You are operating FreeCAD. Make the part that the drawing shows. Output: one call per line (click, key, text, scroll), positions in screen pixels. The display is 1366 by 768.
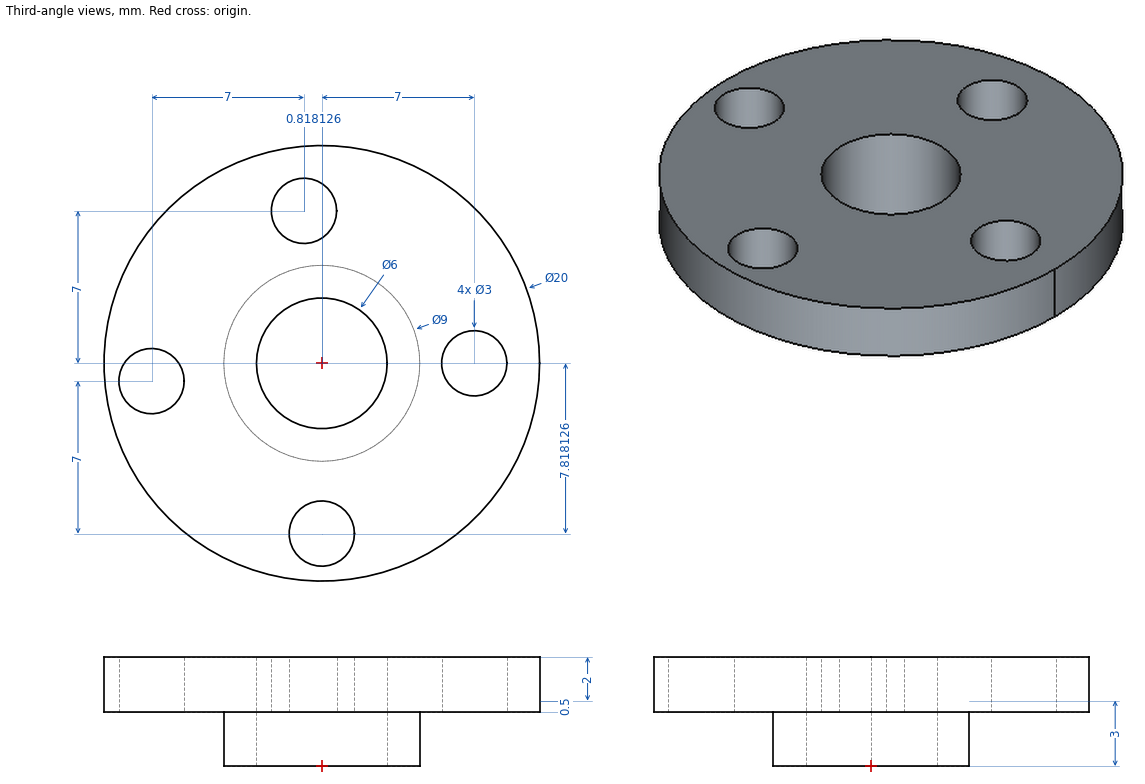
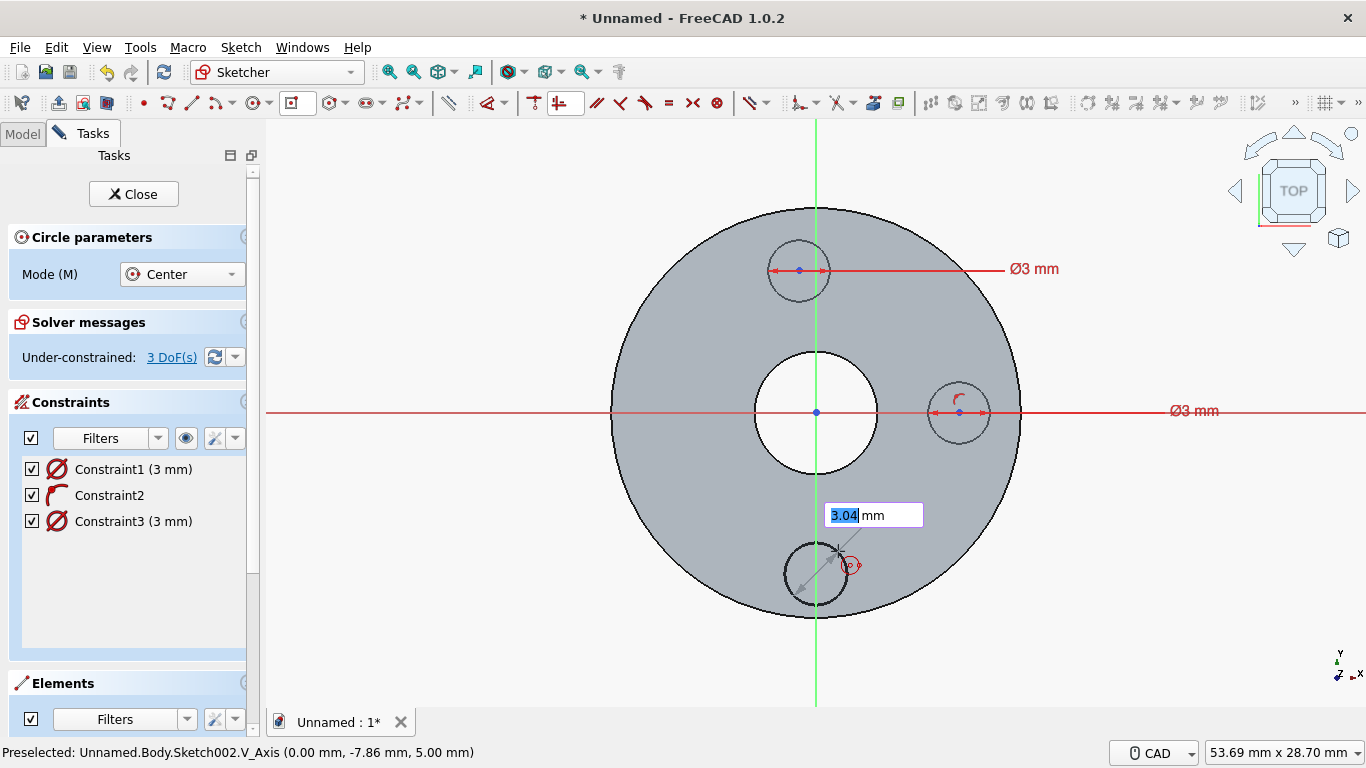
text(3)
key(Return)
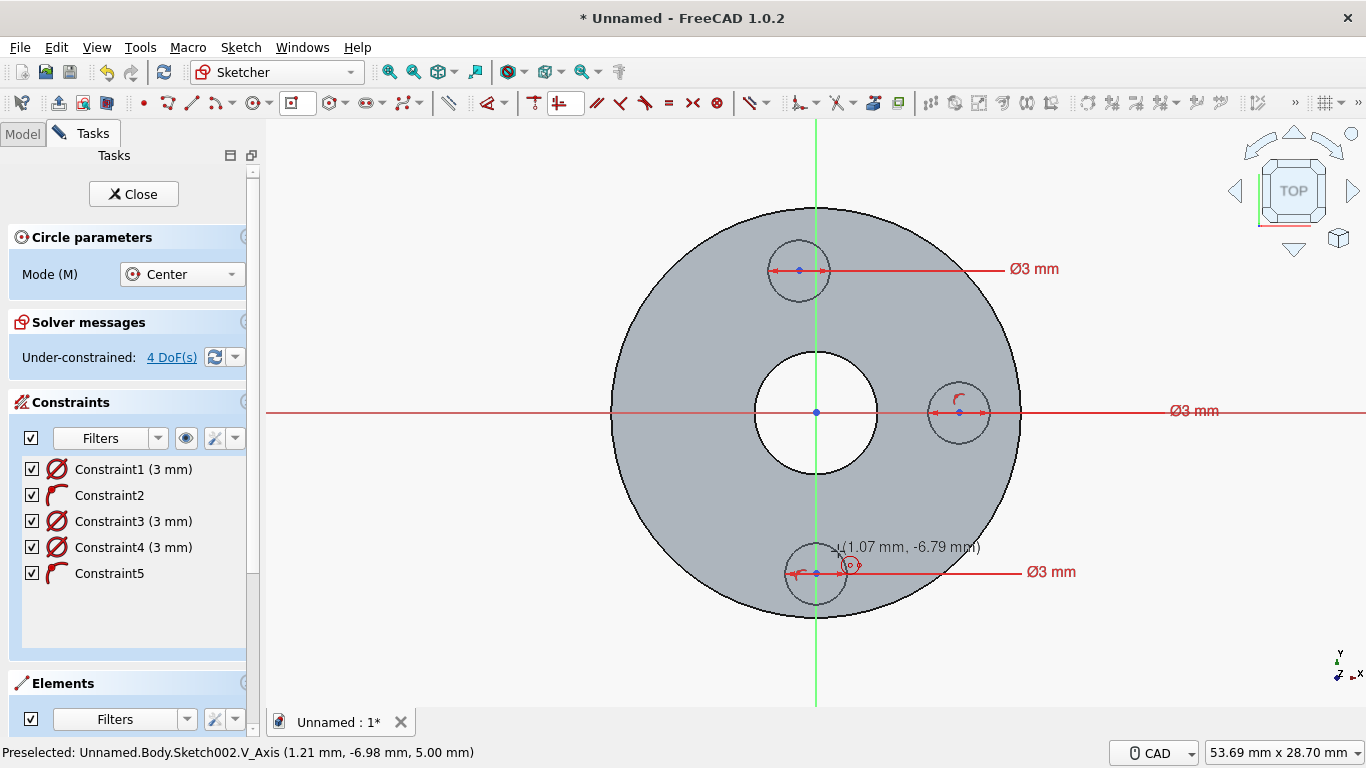
click(656, 430)
move(678, 451)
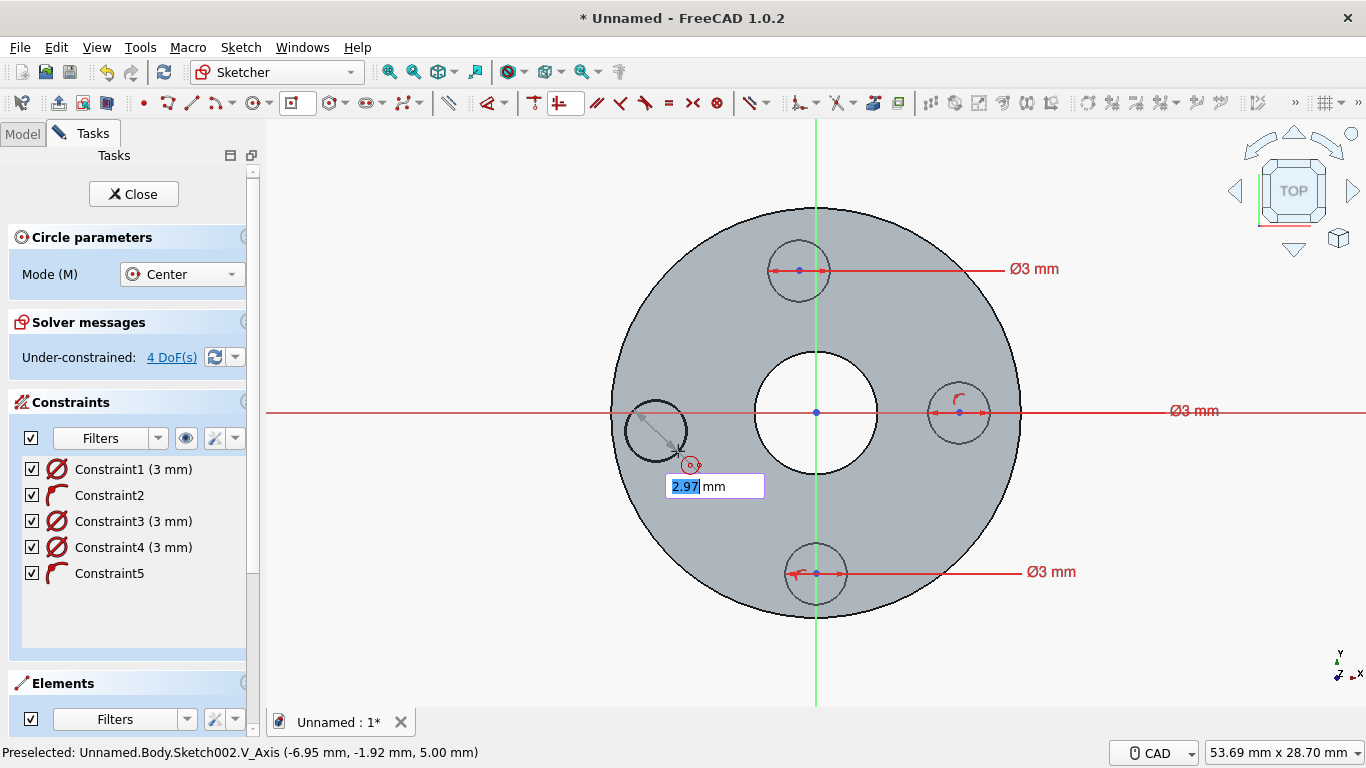
text(3)
key(Return)
key(Escape)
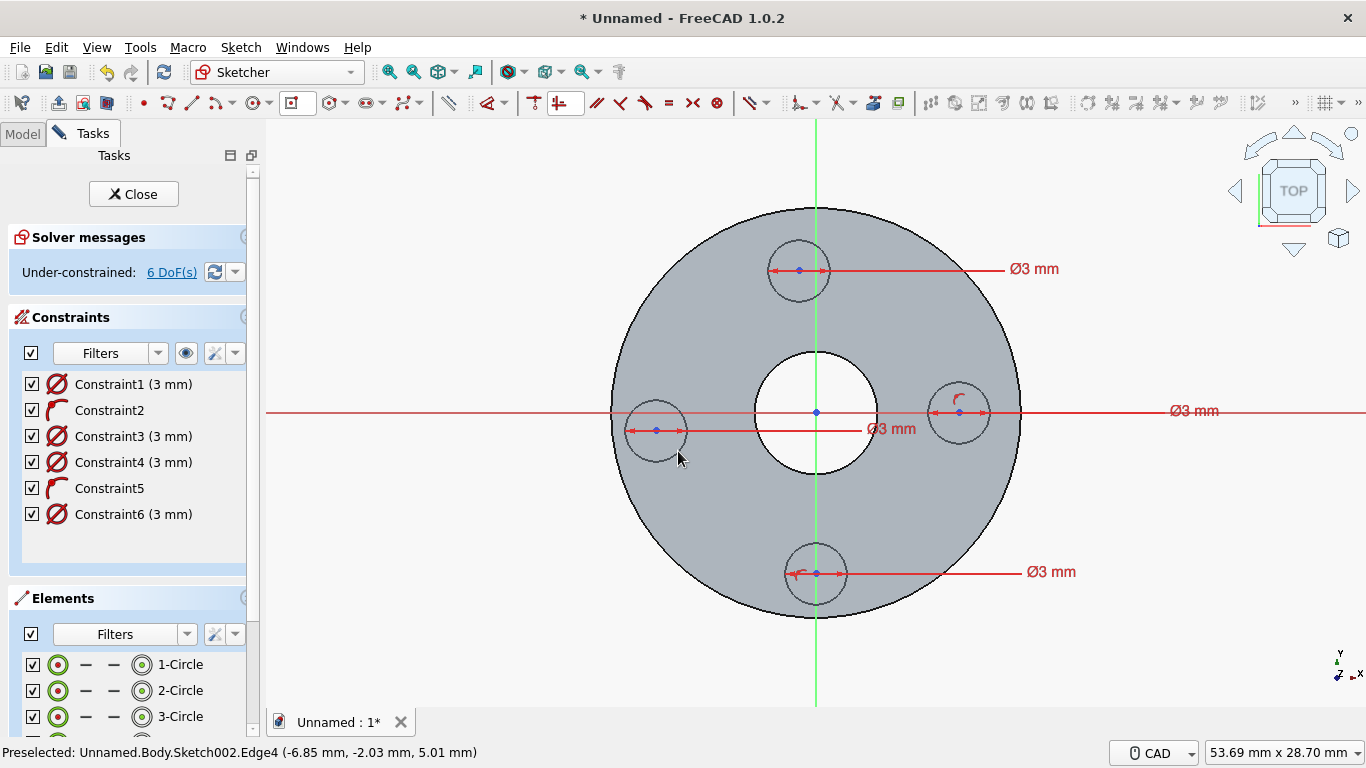
click(959, 413)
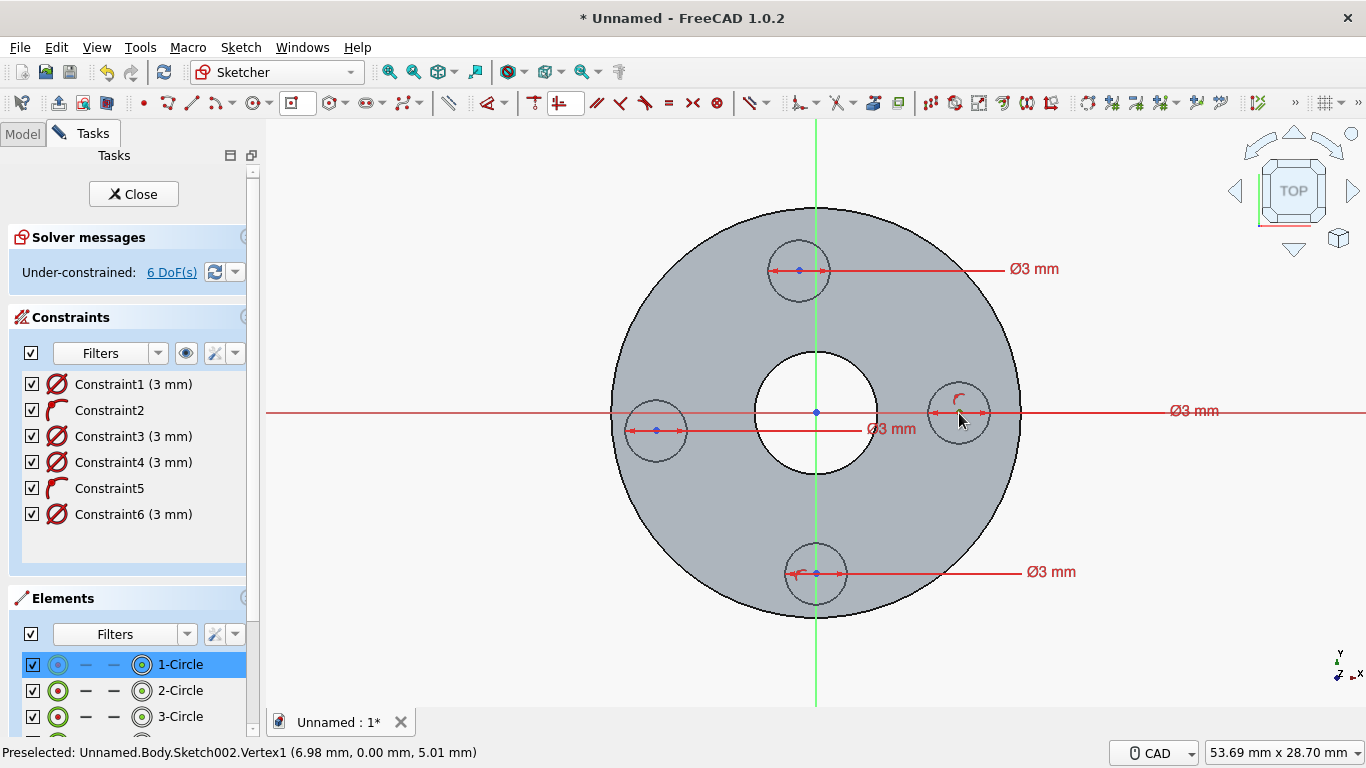
click(506, 104)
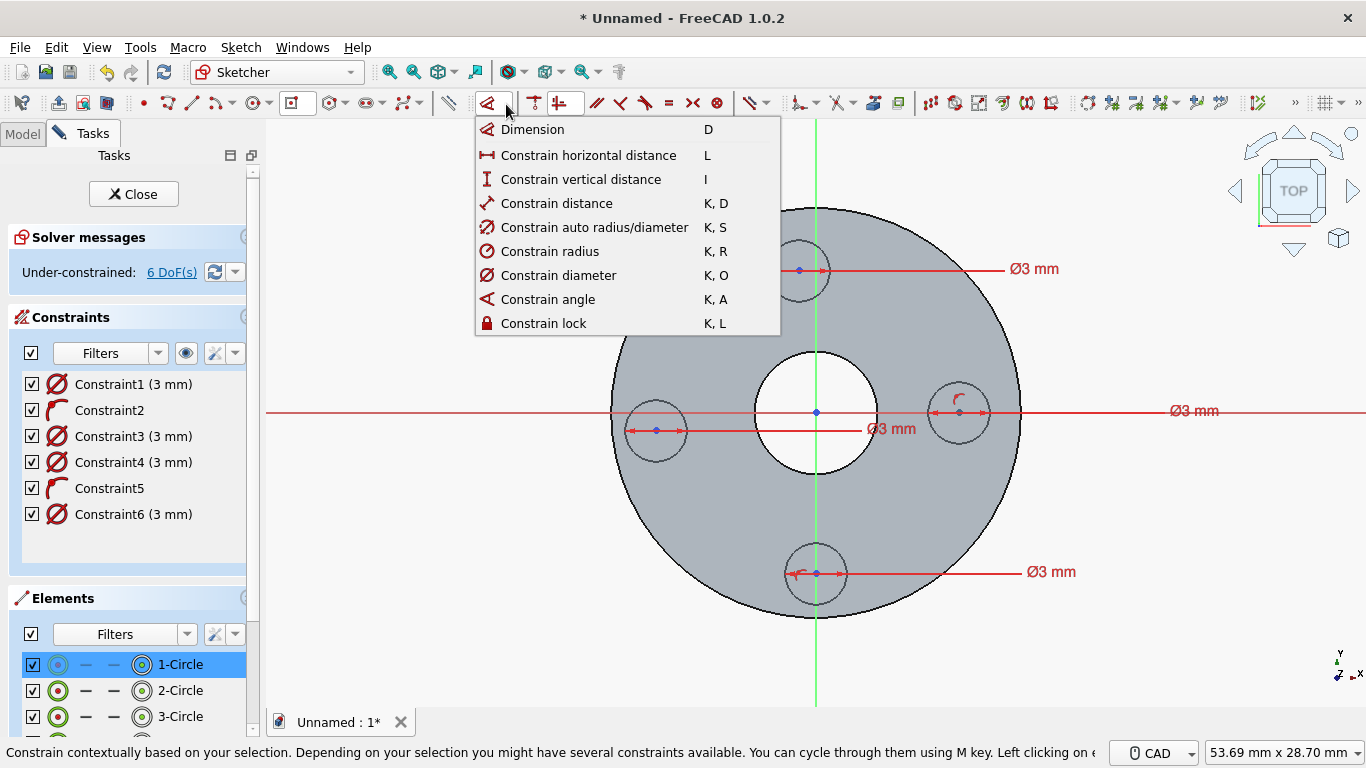
click(628, 155)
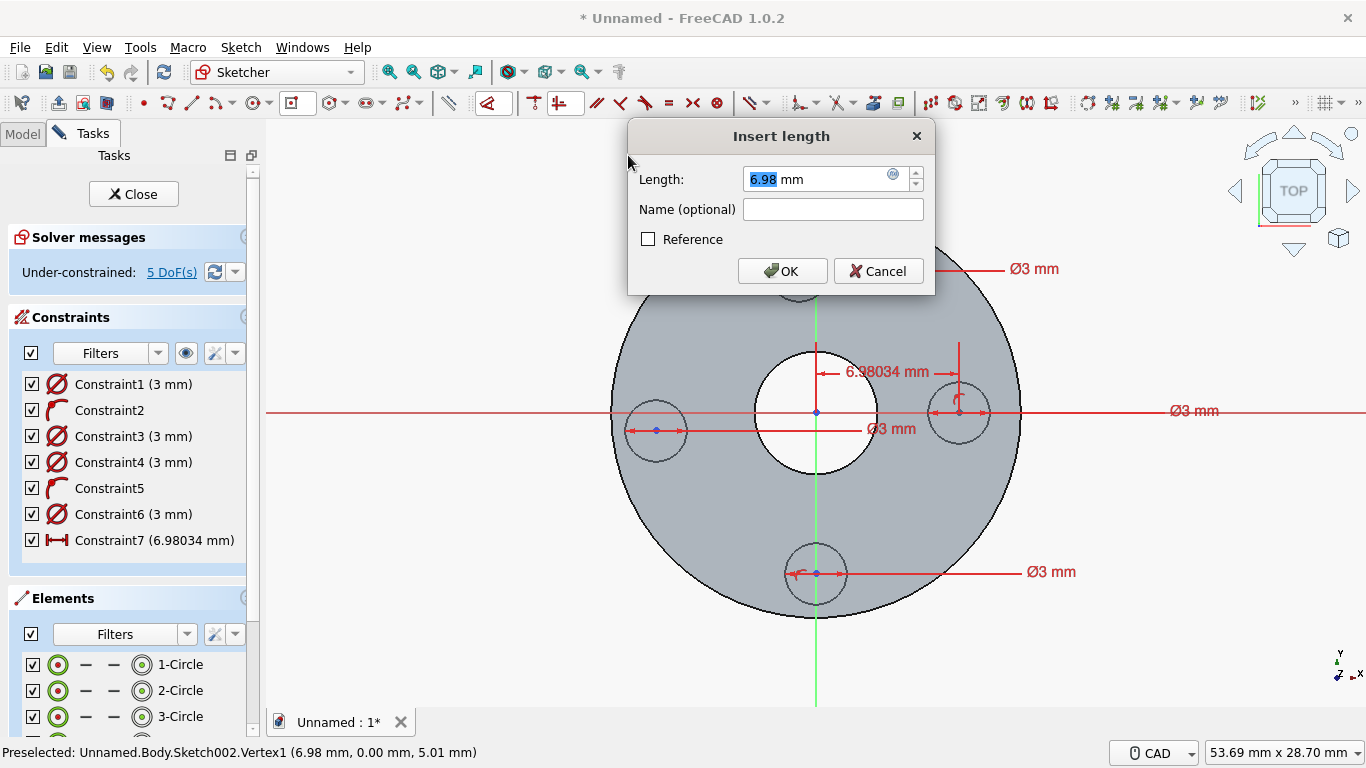
text(7)
key(Return)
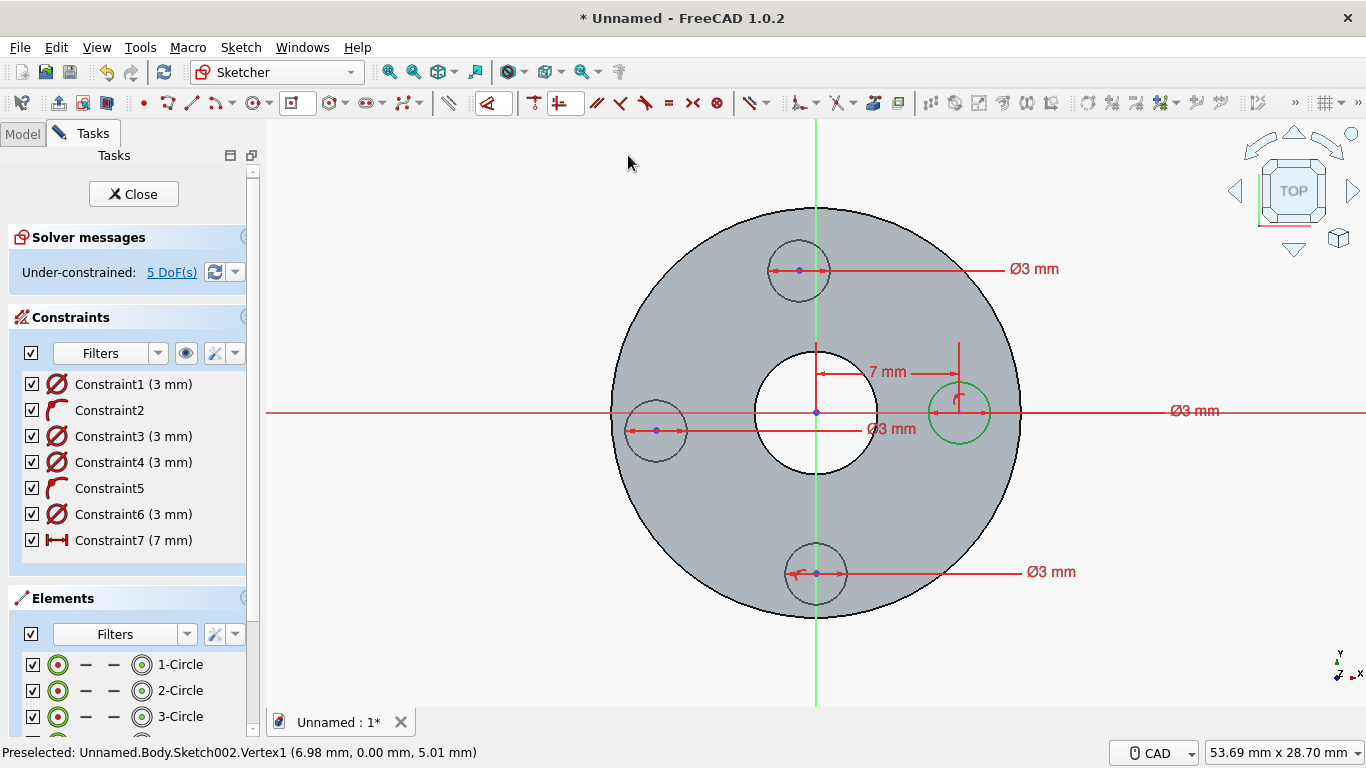
click(799, 271)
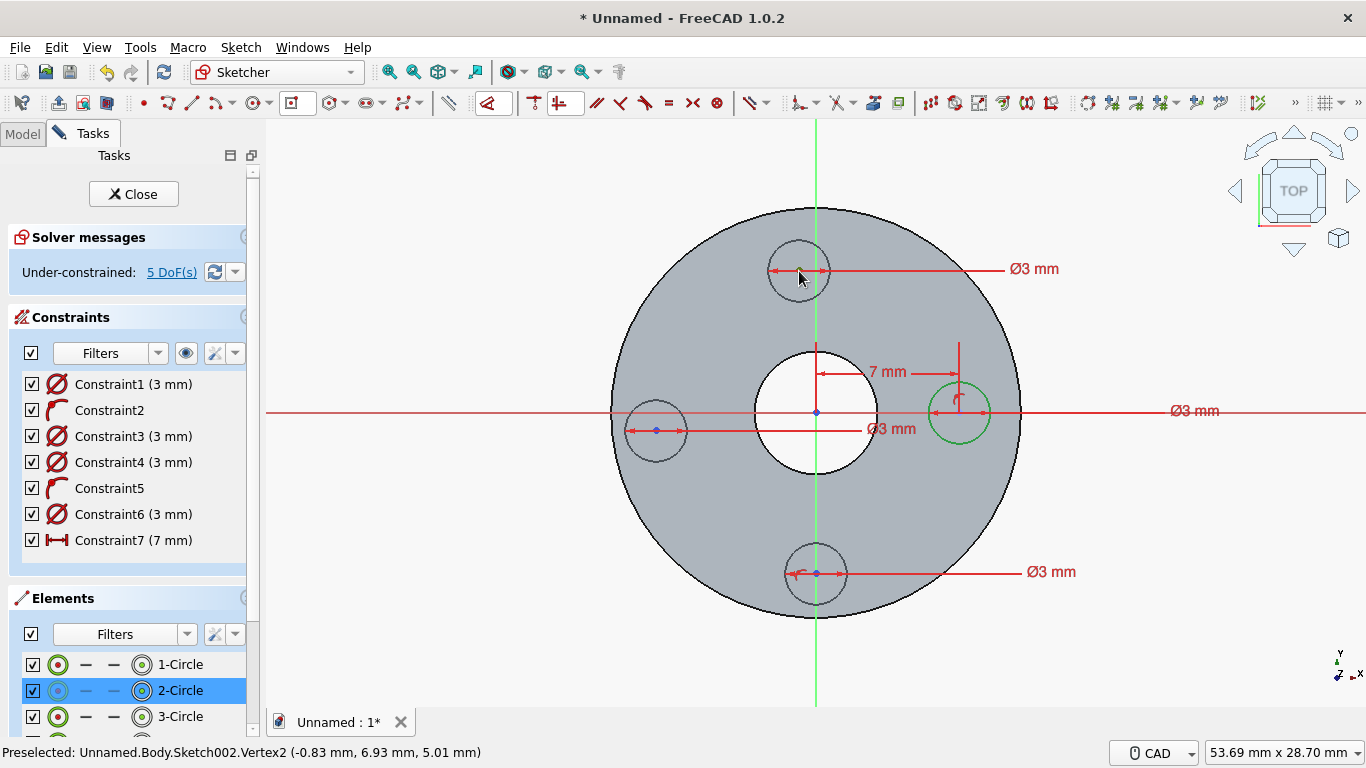
key(i)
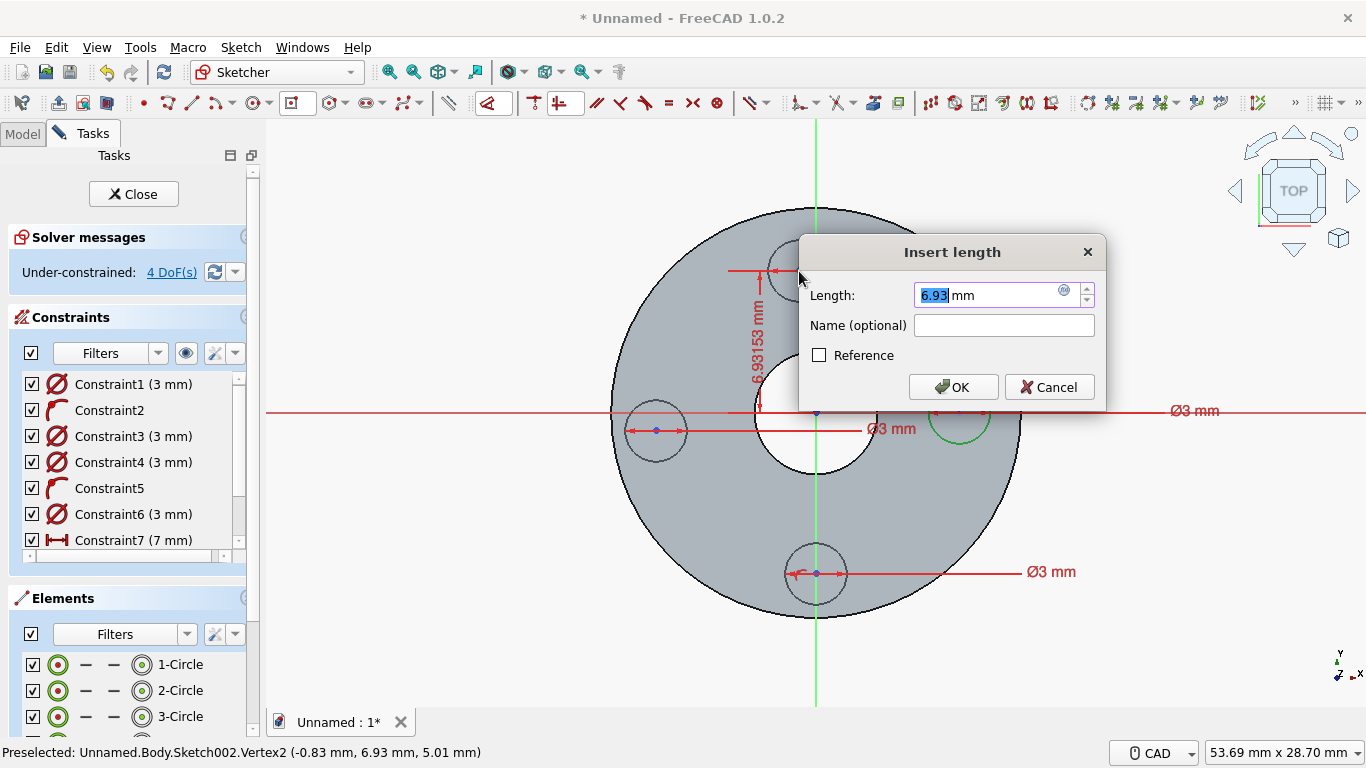
text(7)
key(Return)